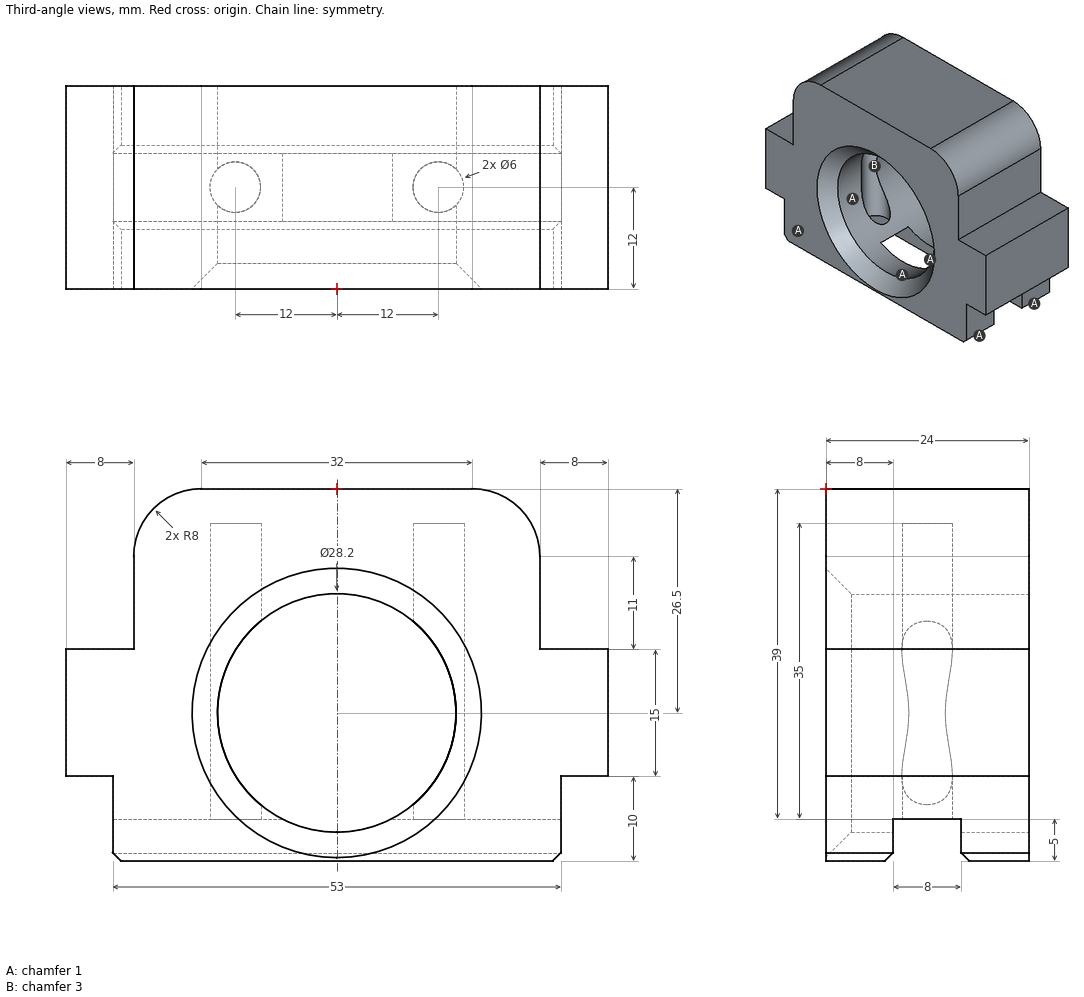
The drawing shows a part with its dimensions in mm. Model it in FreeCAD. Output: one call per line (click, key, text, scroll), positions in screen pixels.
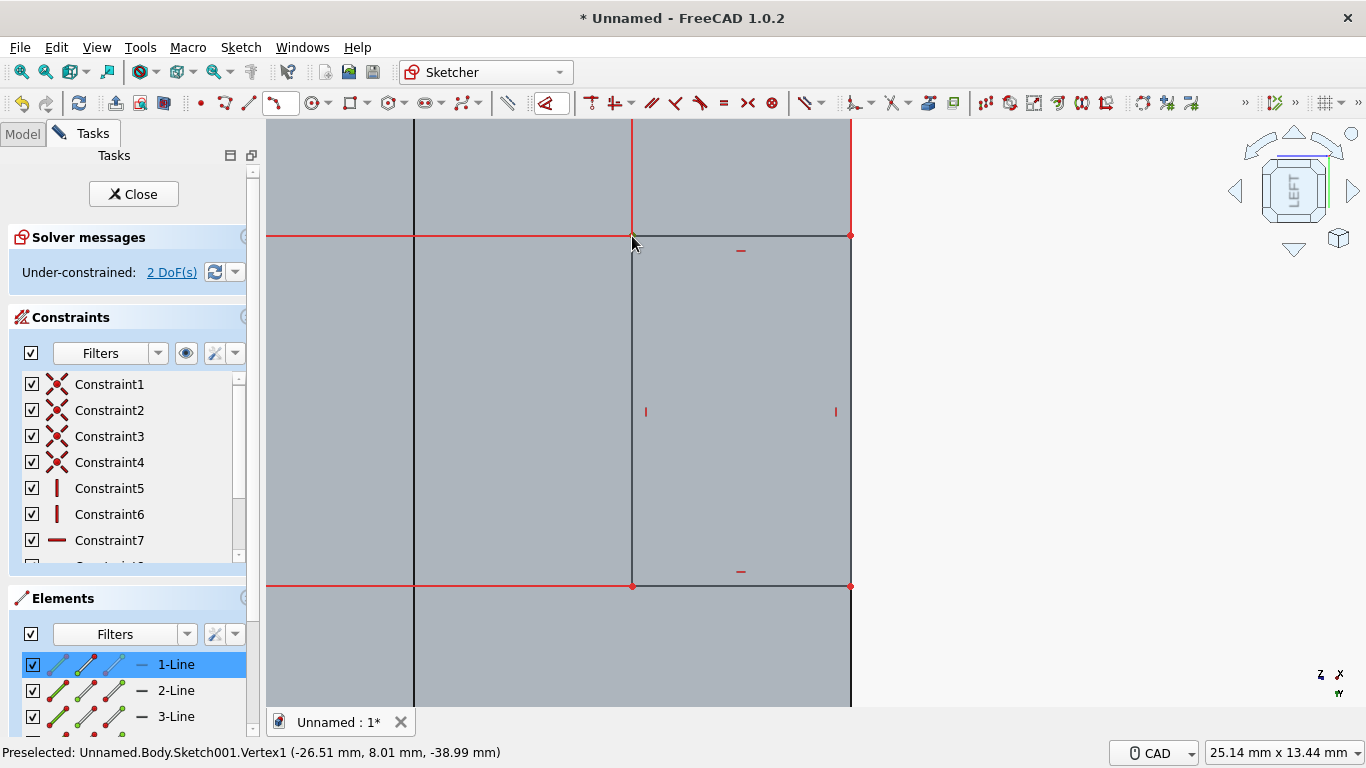
key(i)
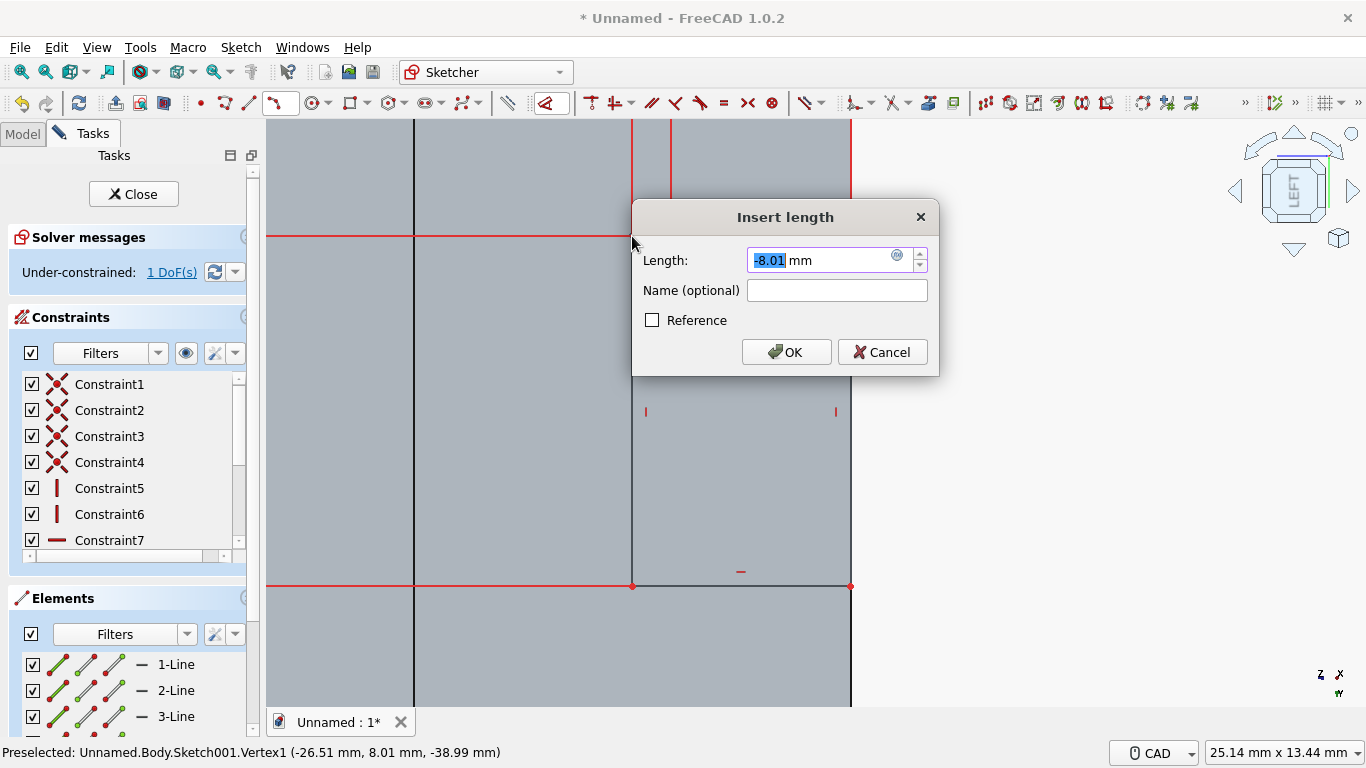
text(-8)
key(Return)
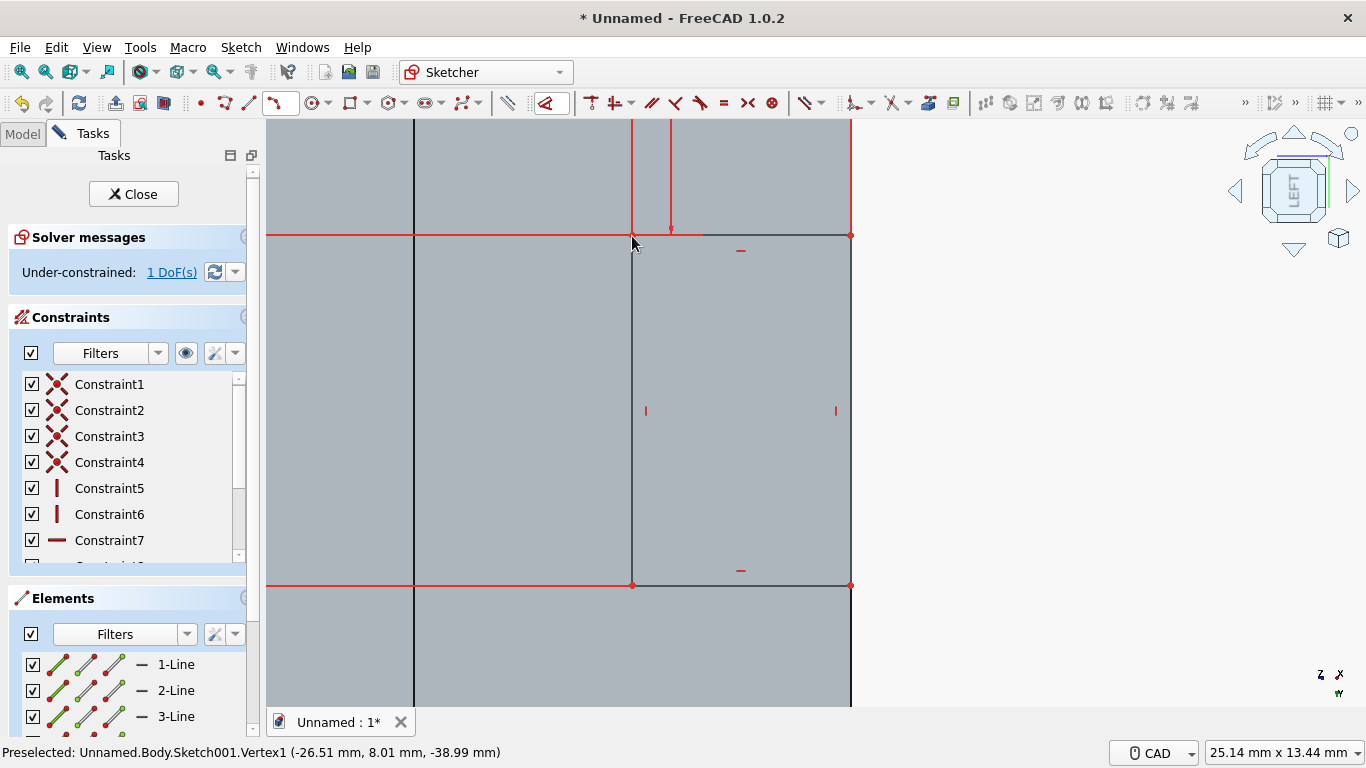
click(632, 235)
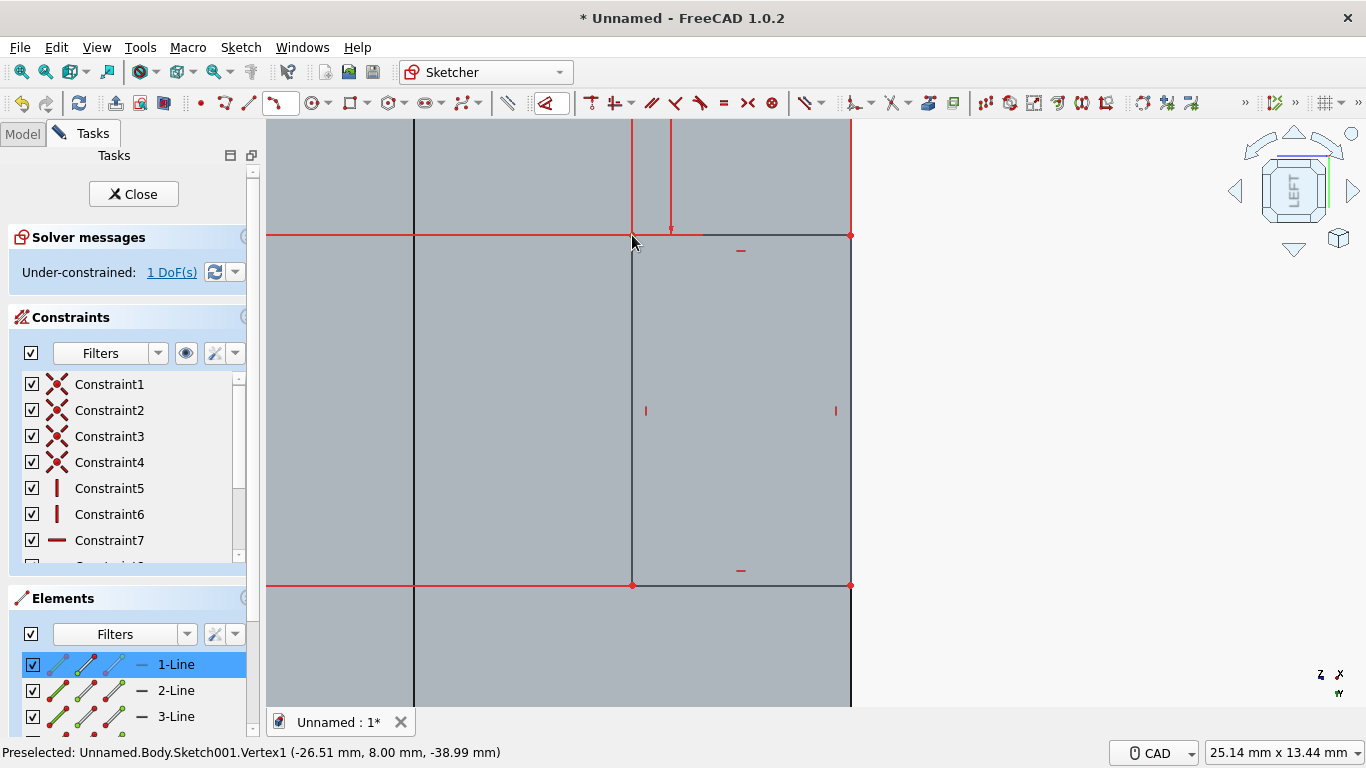
click(564, 104)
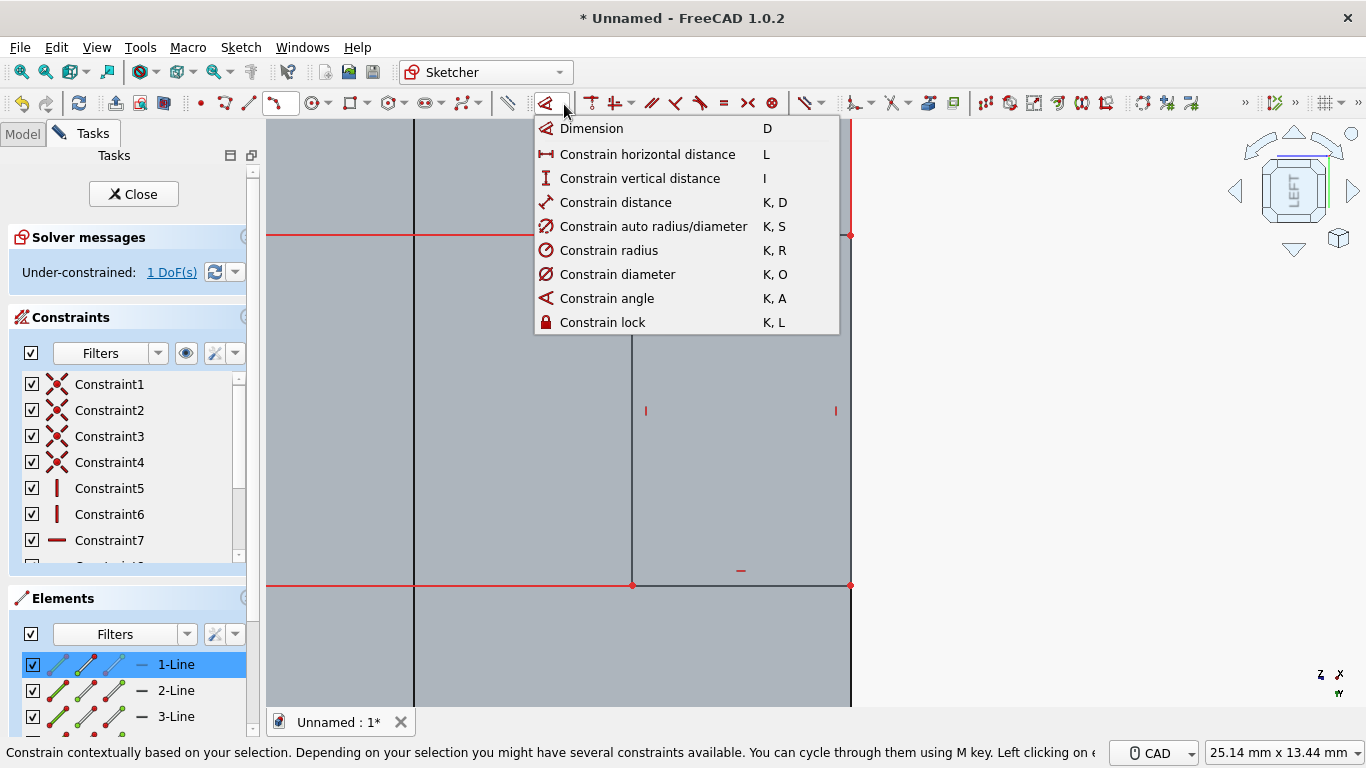
click(687, 154)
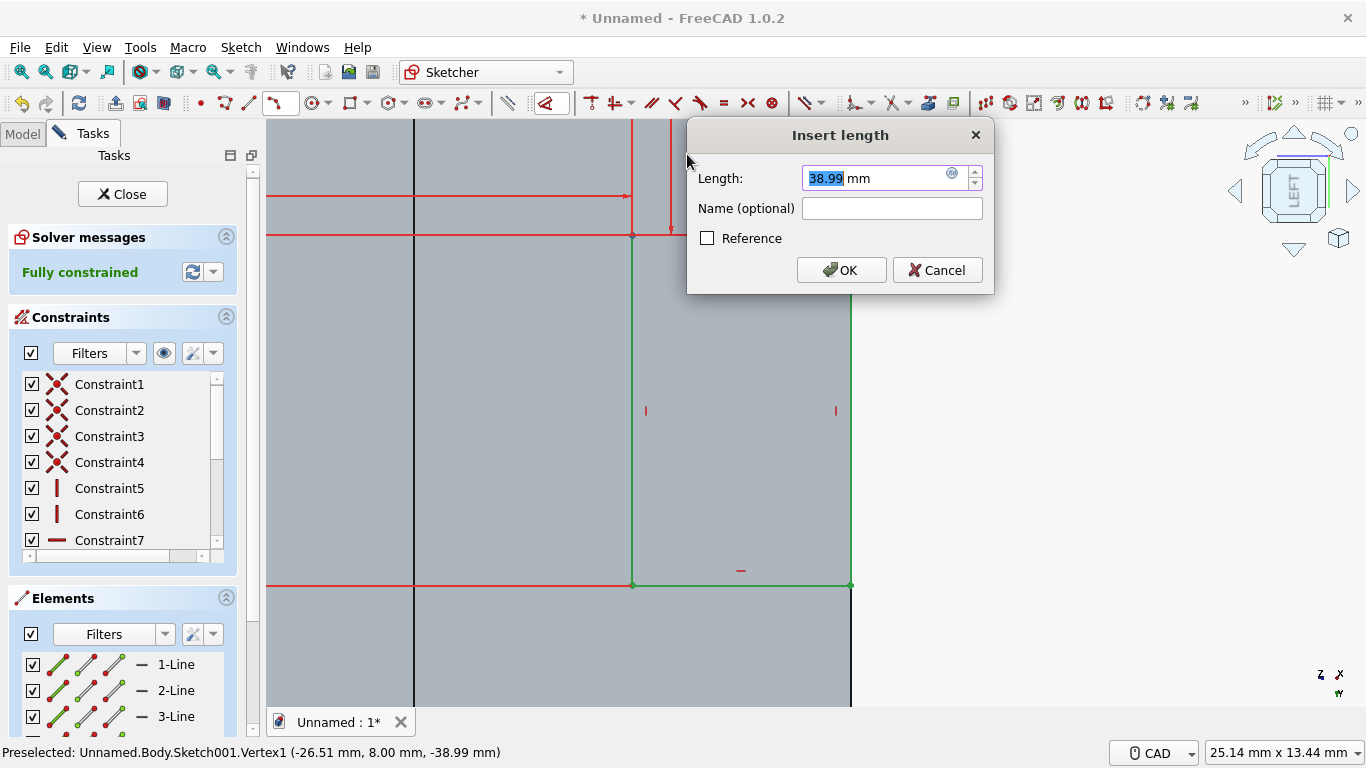
text(39)
key(Return)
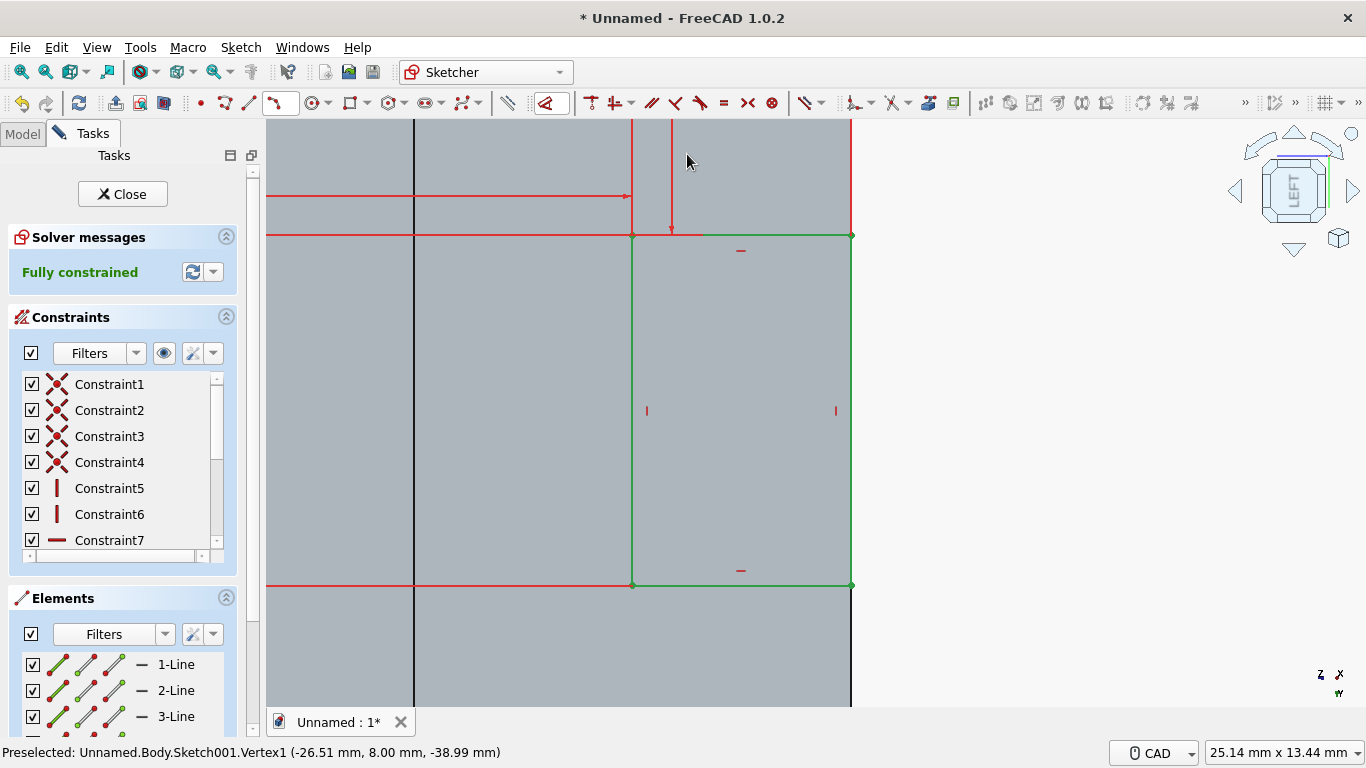
click(123, 194)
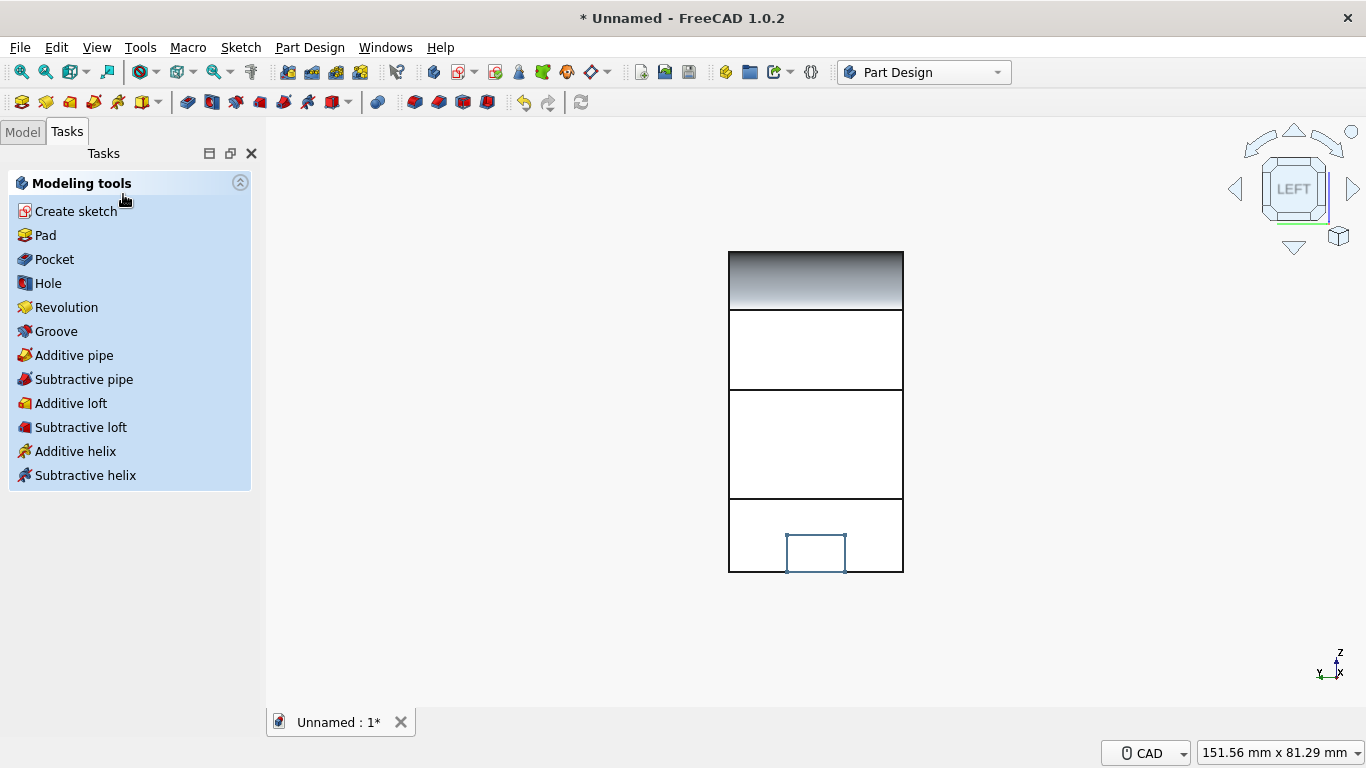
click(188, 102)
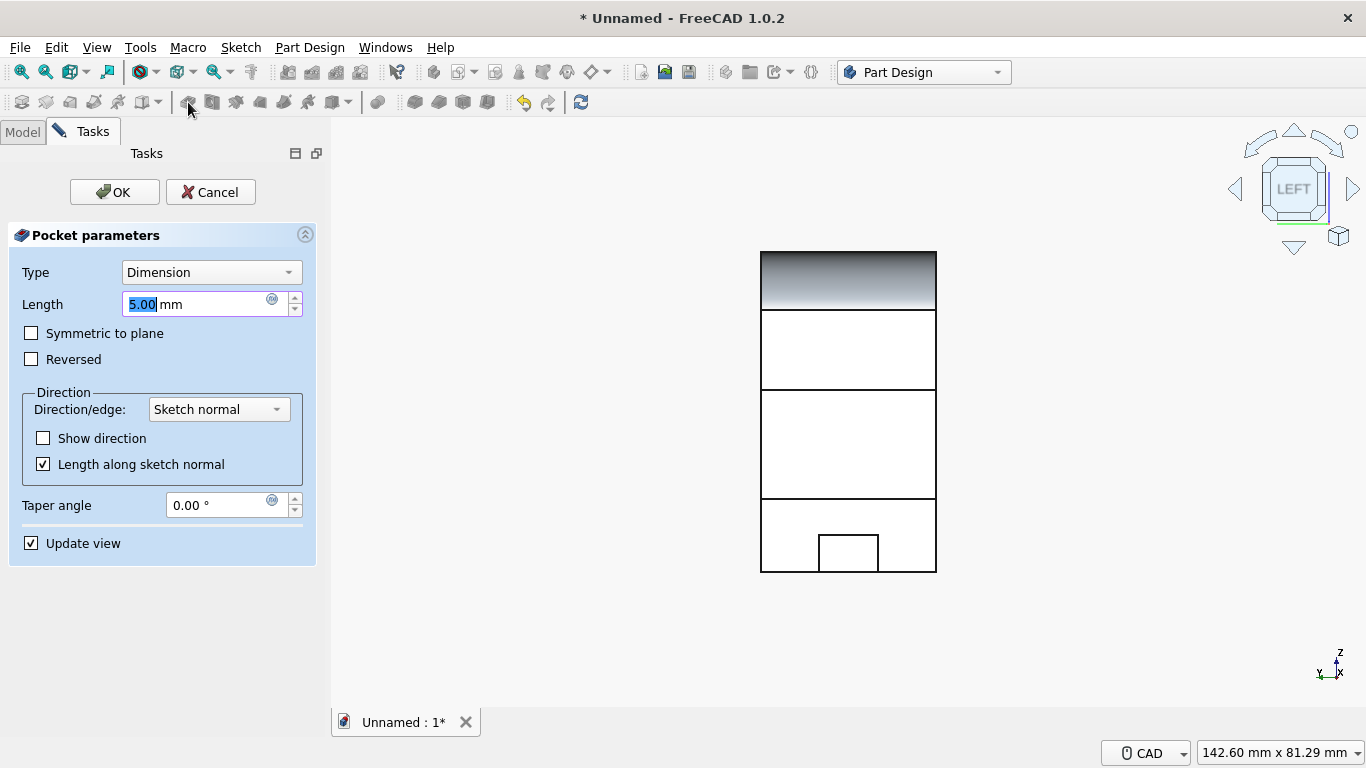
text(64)
key(Tab)